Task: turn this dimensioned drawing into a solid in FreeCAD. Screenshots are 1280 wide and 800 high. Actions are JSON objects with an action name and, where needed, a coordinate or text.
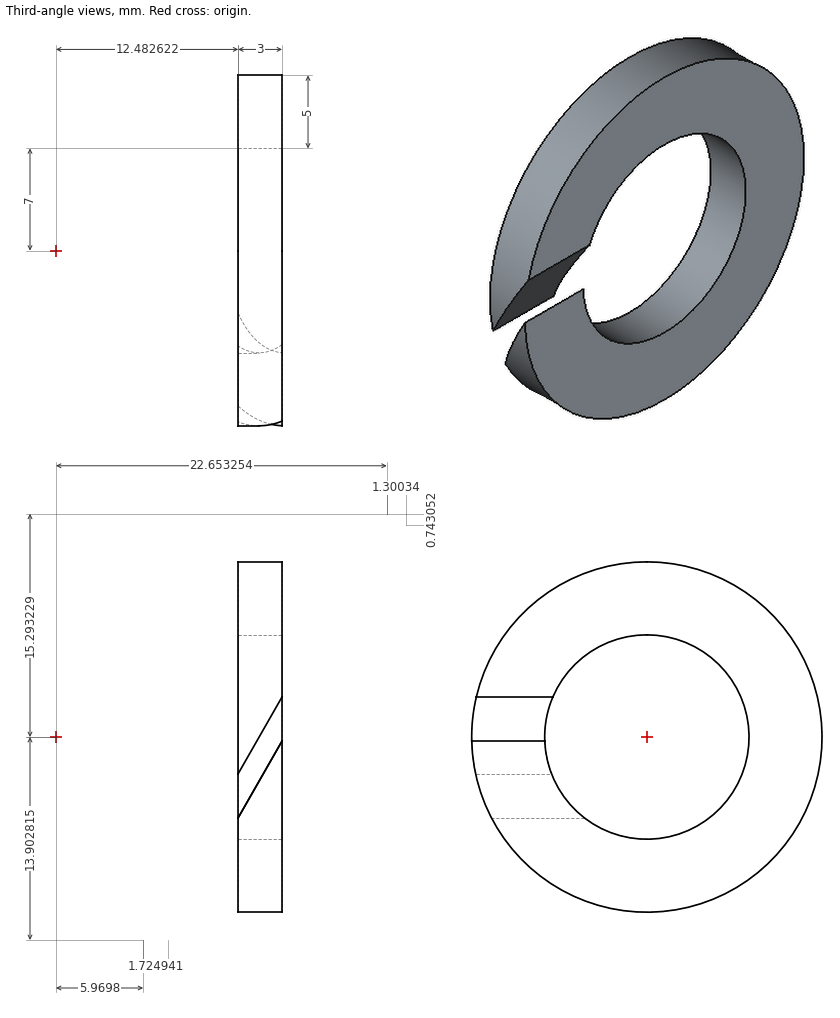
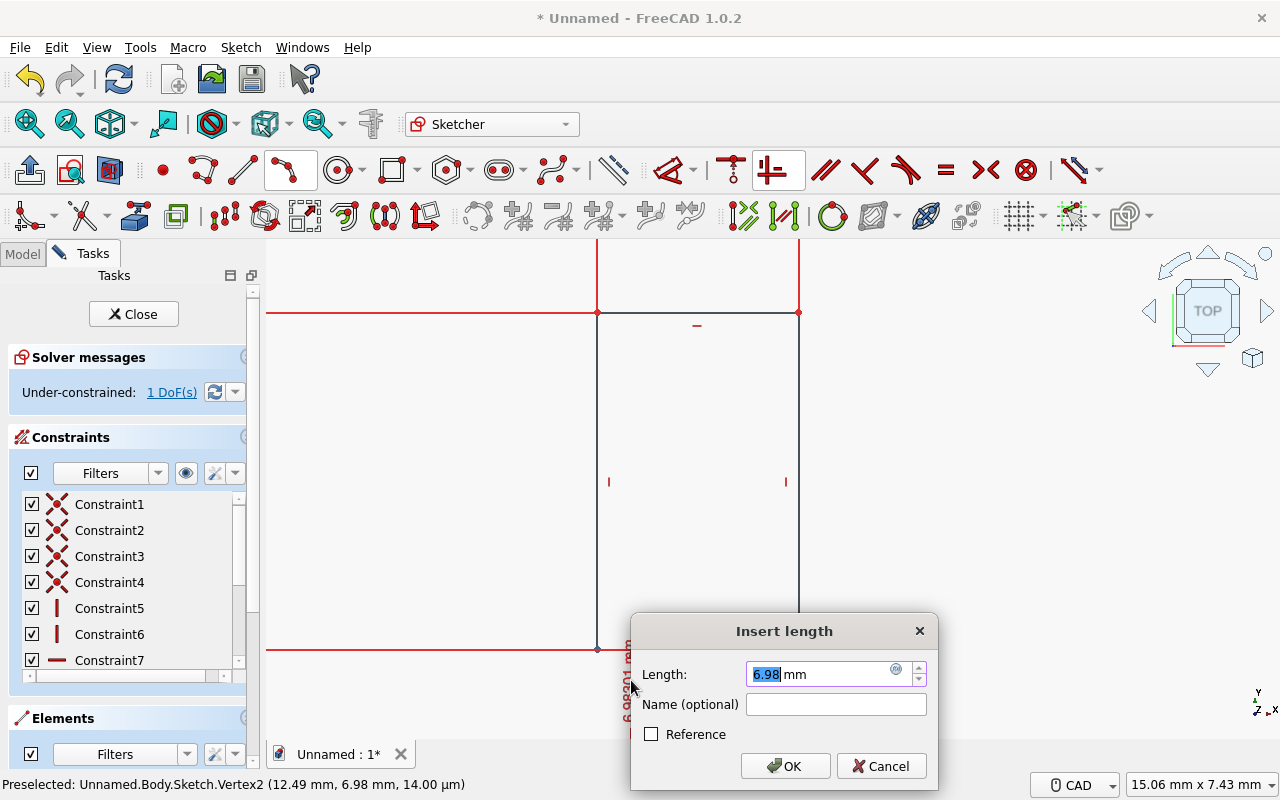
{"action": "type", "text": "7"}
{"action": "key", "text": "Return"}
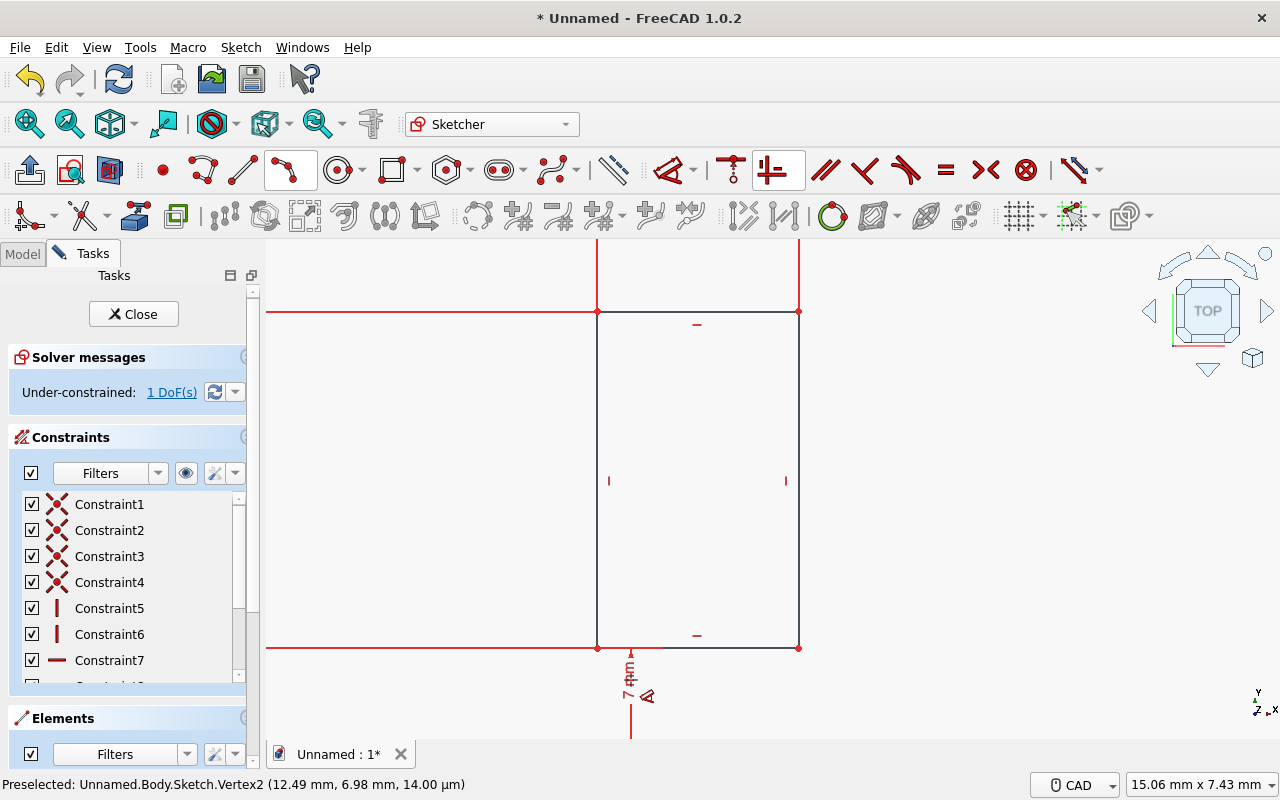
{"action": "left_click", "coordinate": [597, 312]}
{"action": "left_click", "coordinate": [446, 278]}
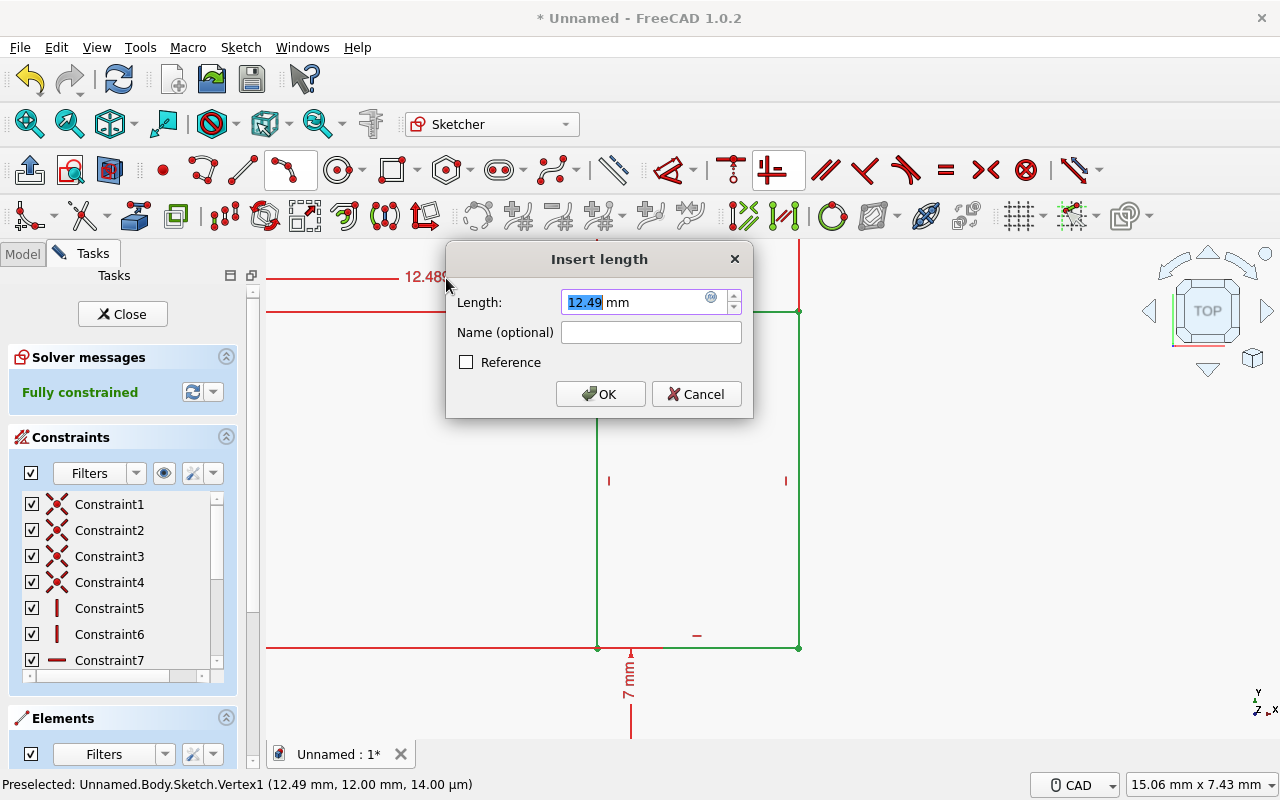
{"action": "type", "text": "12.482622"}
{"action": "key", "text": "Return"}
{"action": "key", "text": "Escape"}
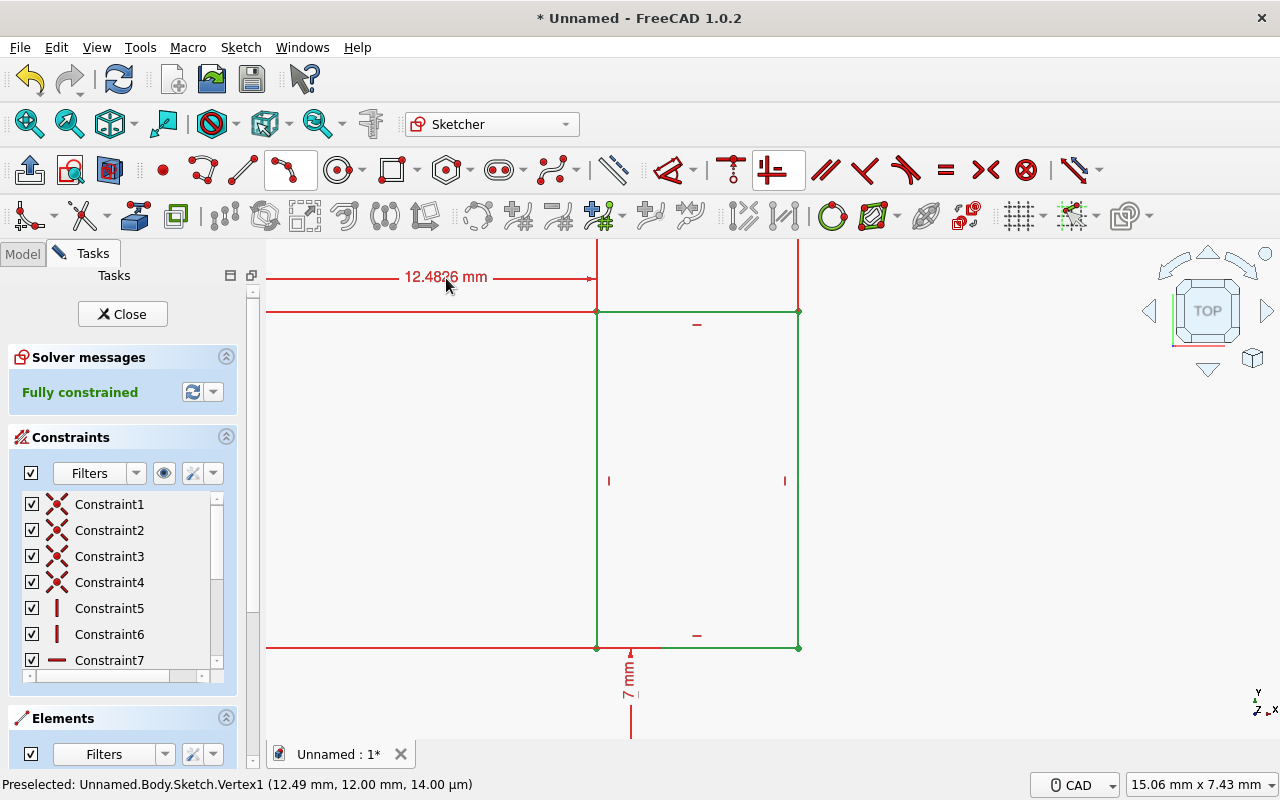
{"action": "left_click", "coordinate": [123, 314]}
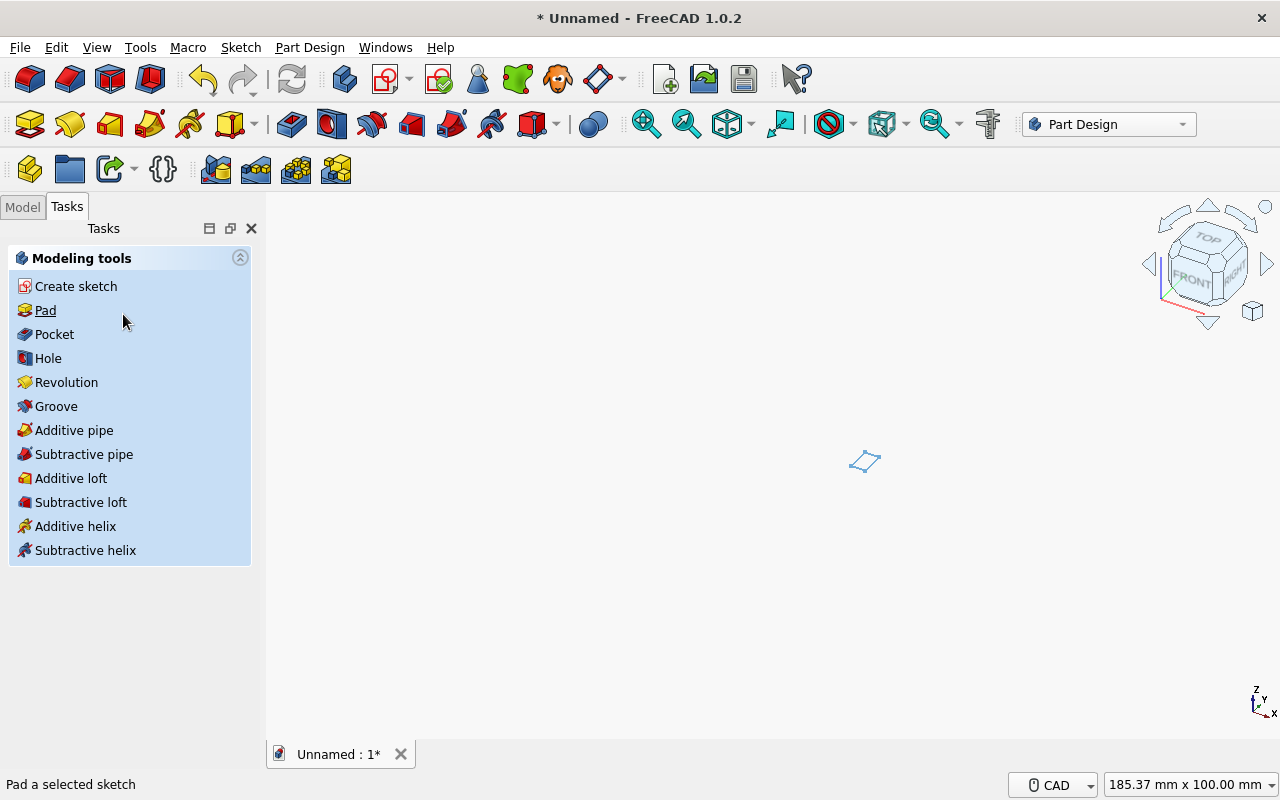
{"action": "left_click", "coordinate": [70, 124]}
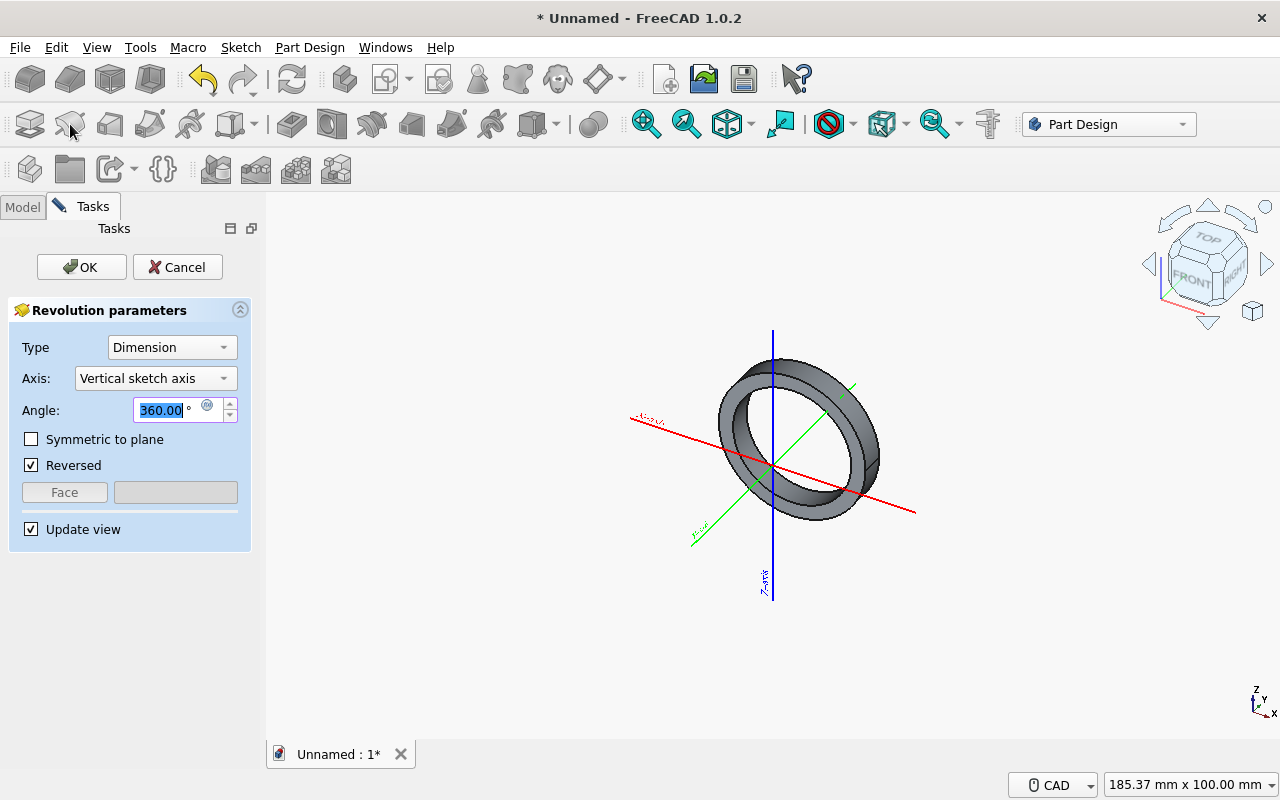
{"action": "left_click", "coordinate": [156, 378]}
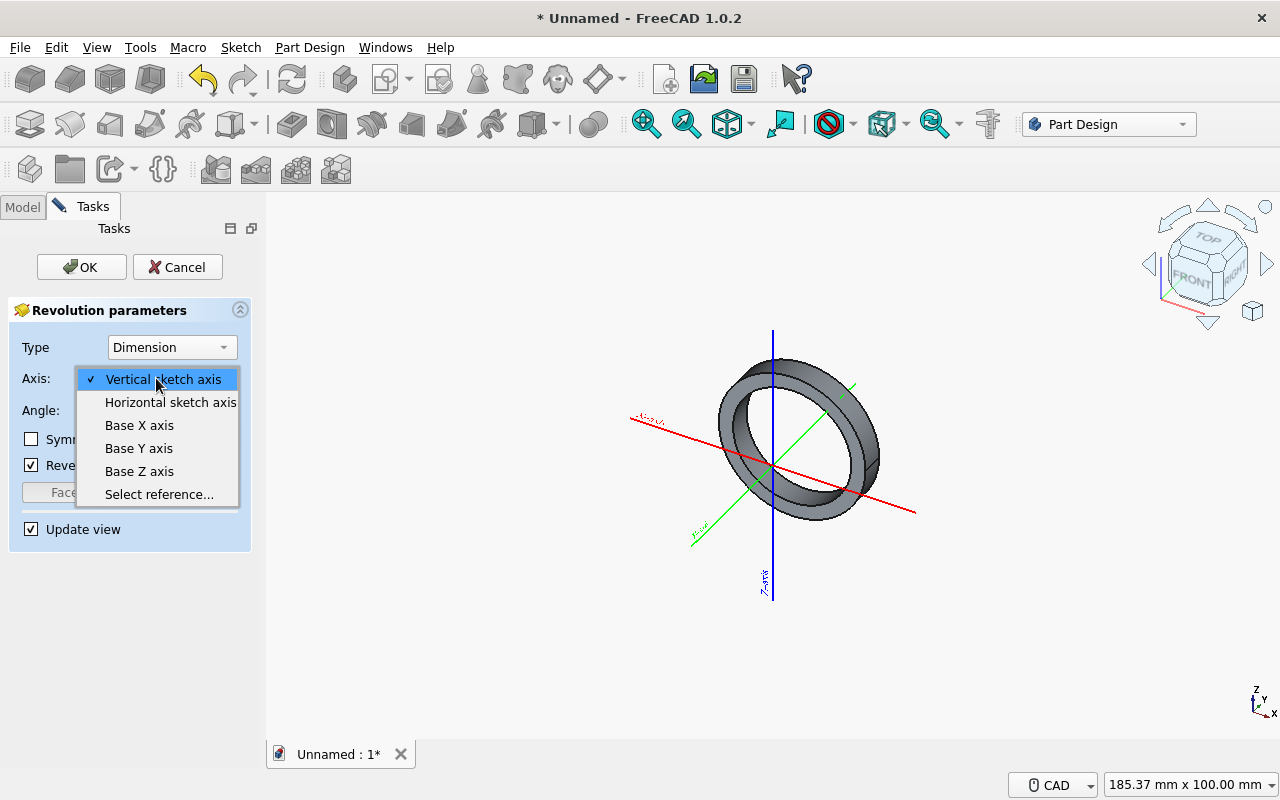
{"action": "left_click", "coordinate": [156, 402]}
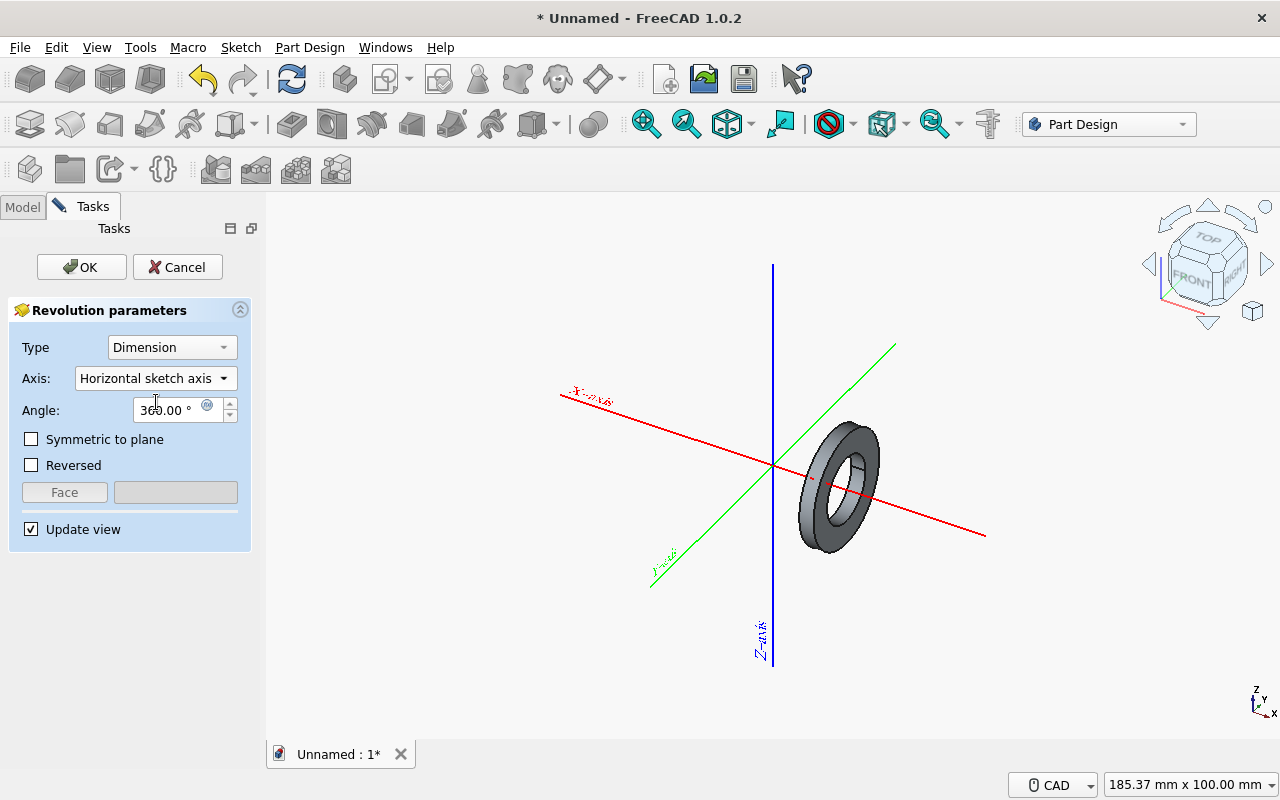
{"action": "left_click", "coordinate": [82, 267]}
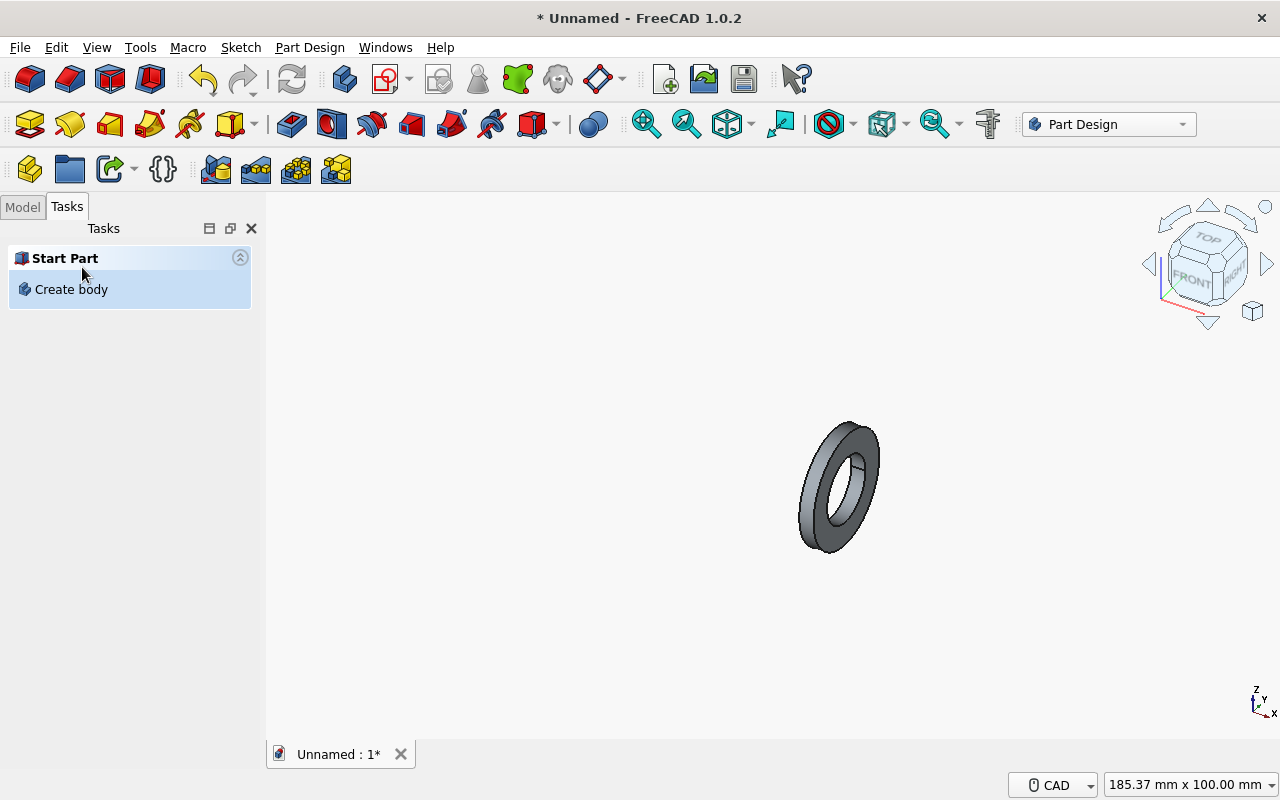
{"action": "key", "text": "v f"}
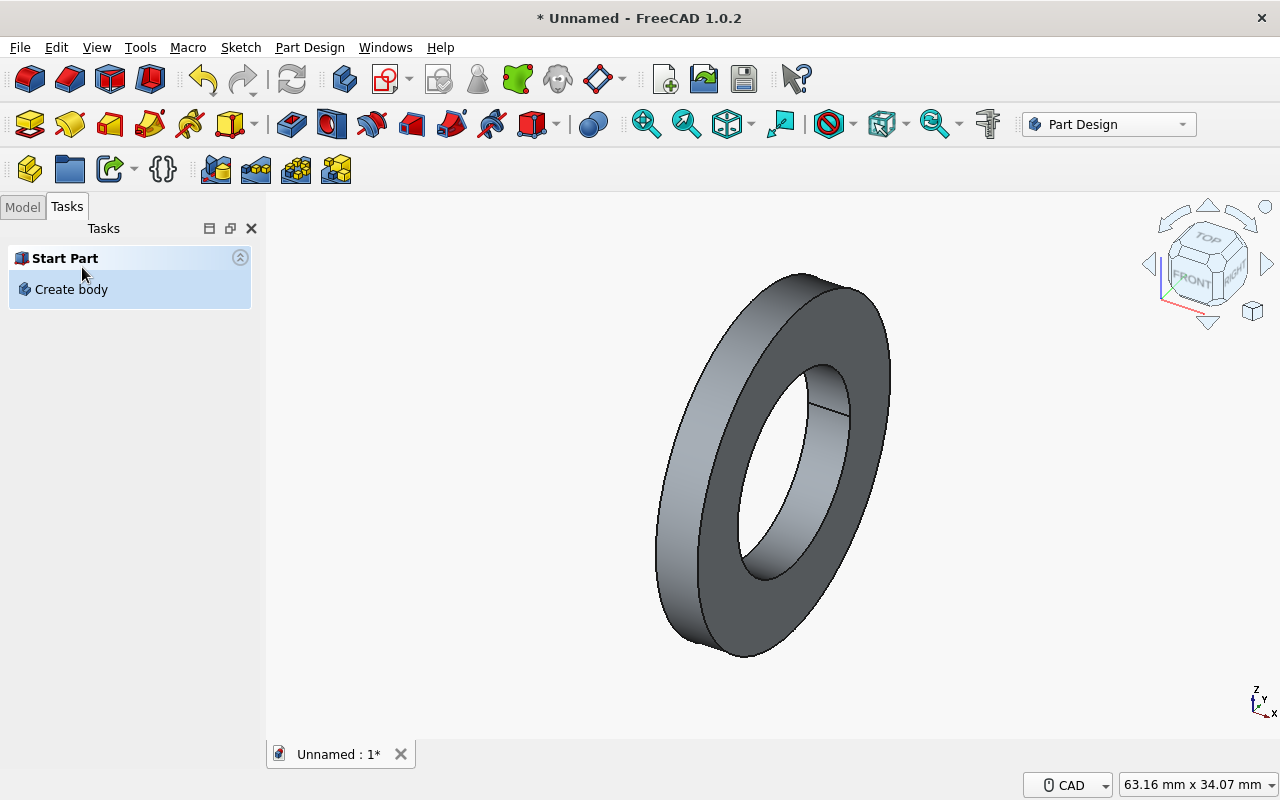
{"action": "left_click", "coordinate": [386, 80]}